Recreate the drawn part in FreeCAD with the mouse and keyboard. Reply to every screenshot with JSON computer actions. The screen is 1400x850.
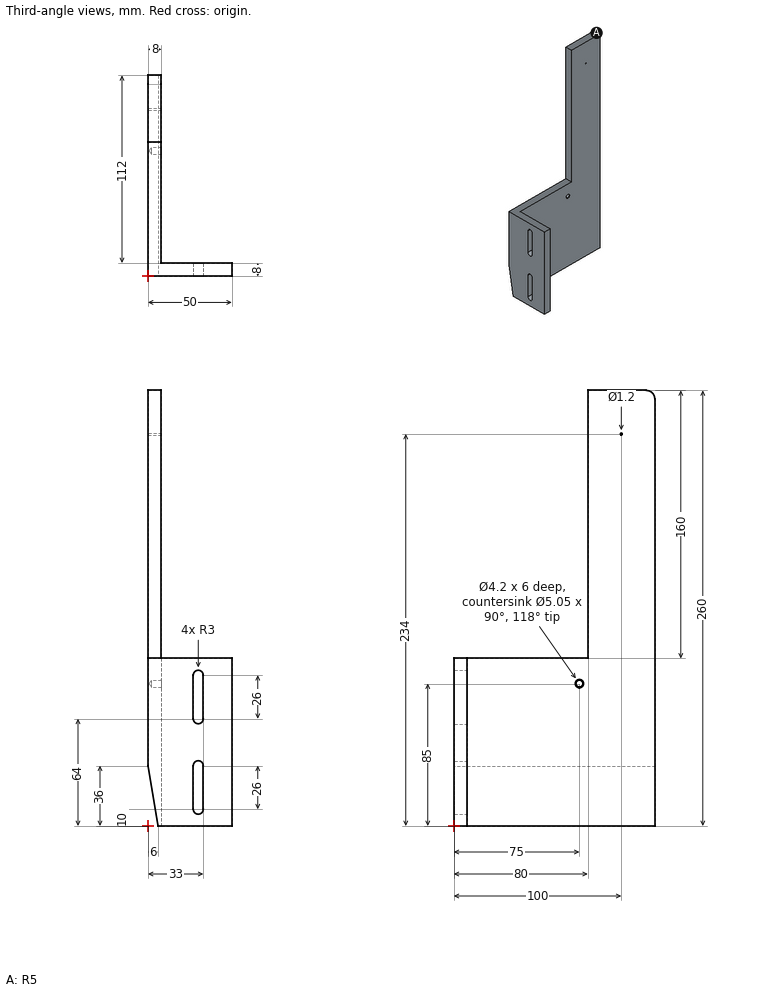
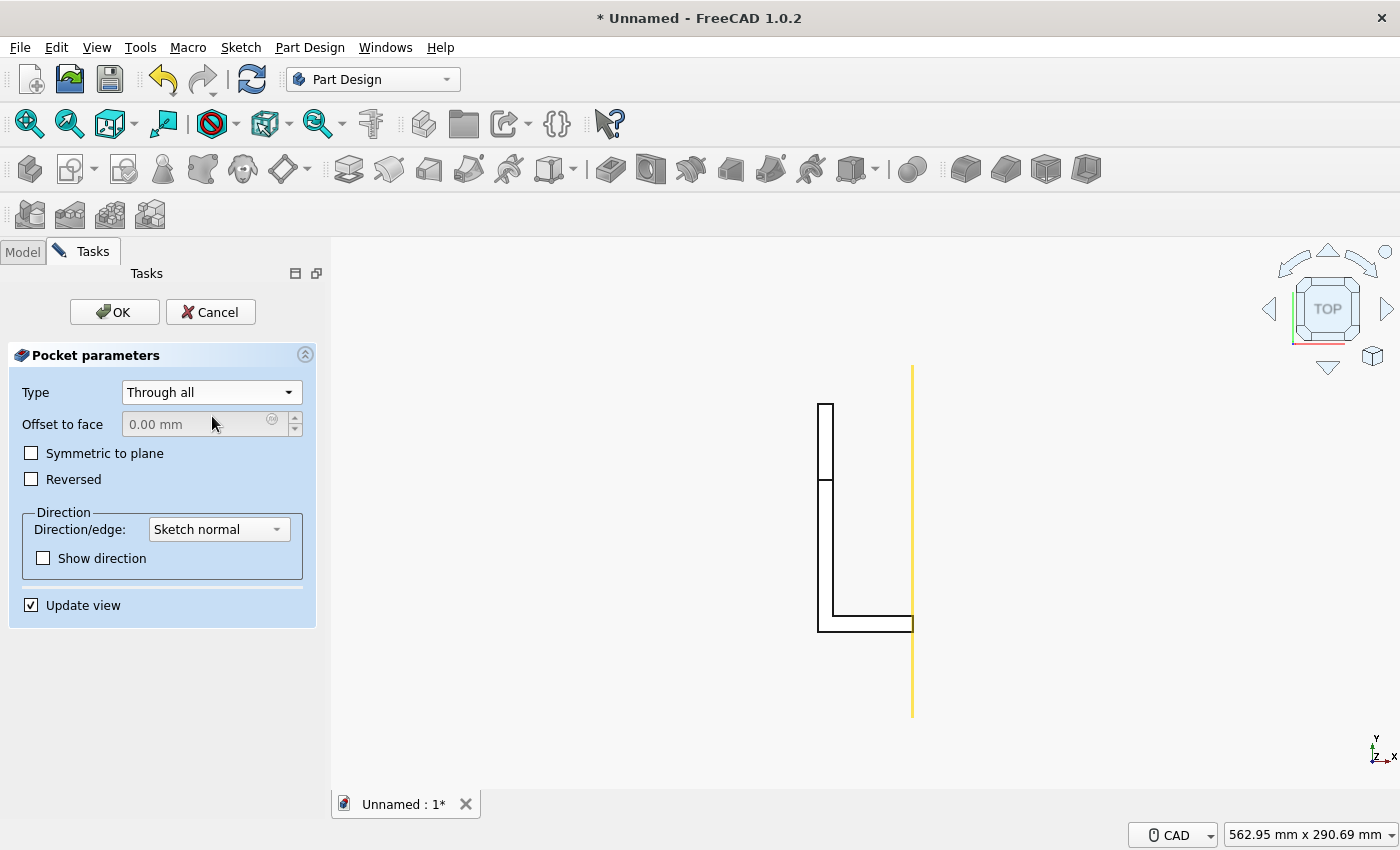
{"action": "left_click", "coordinate": [115, 312]}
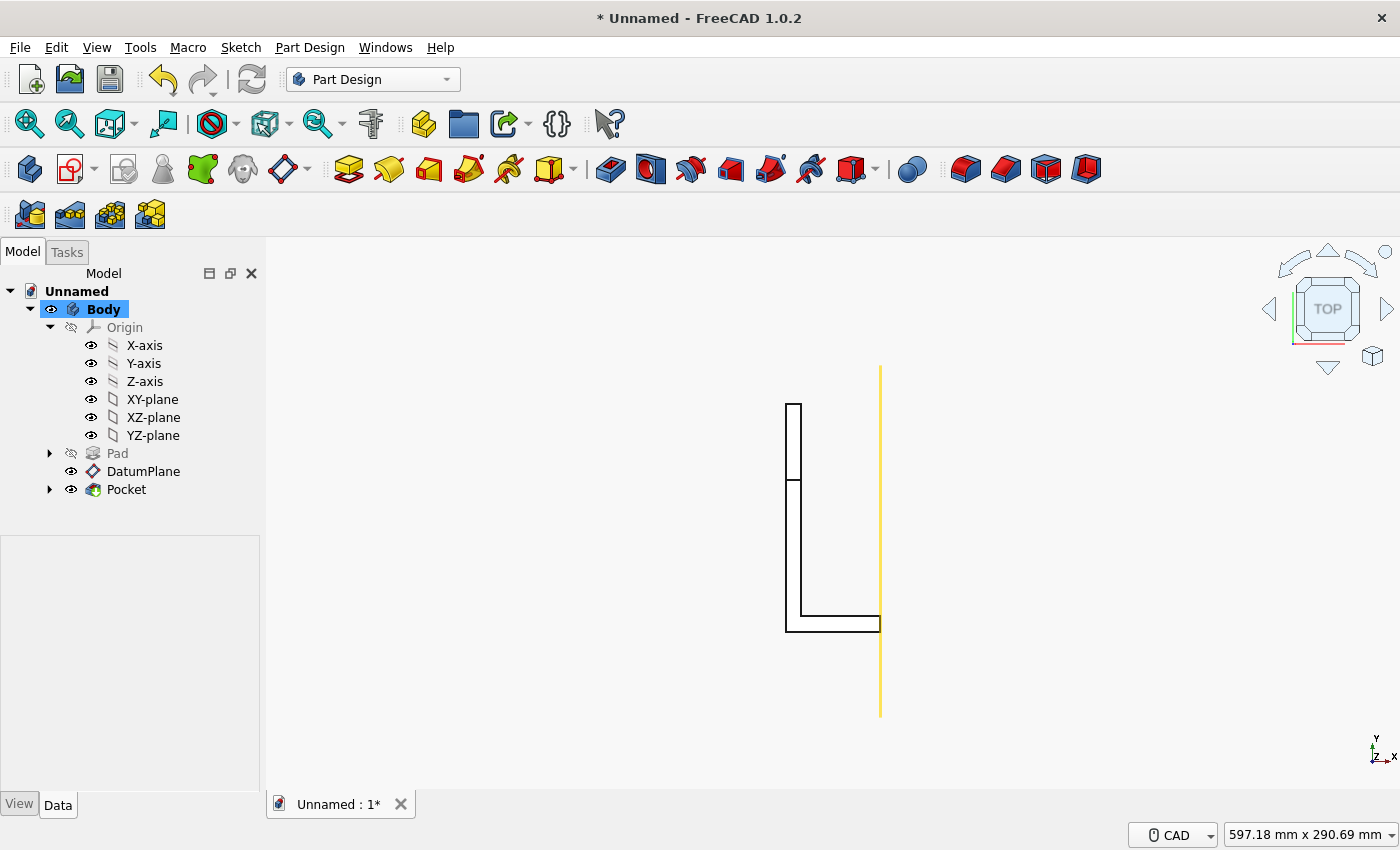
{"action": "left_click", "coordinate": [116, 471]}
{"action": "key", "text": "space"}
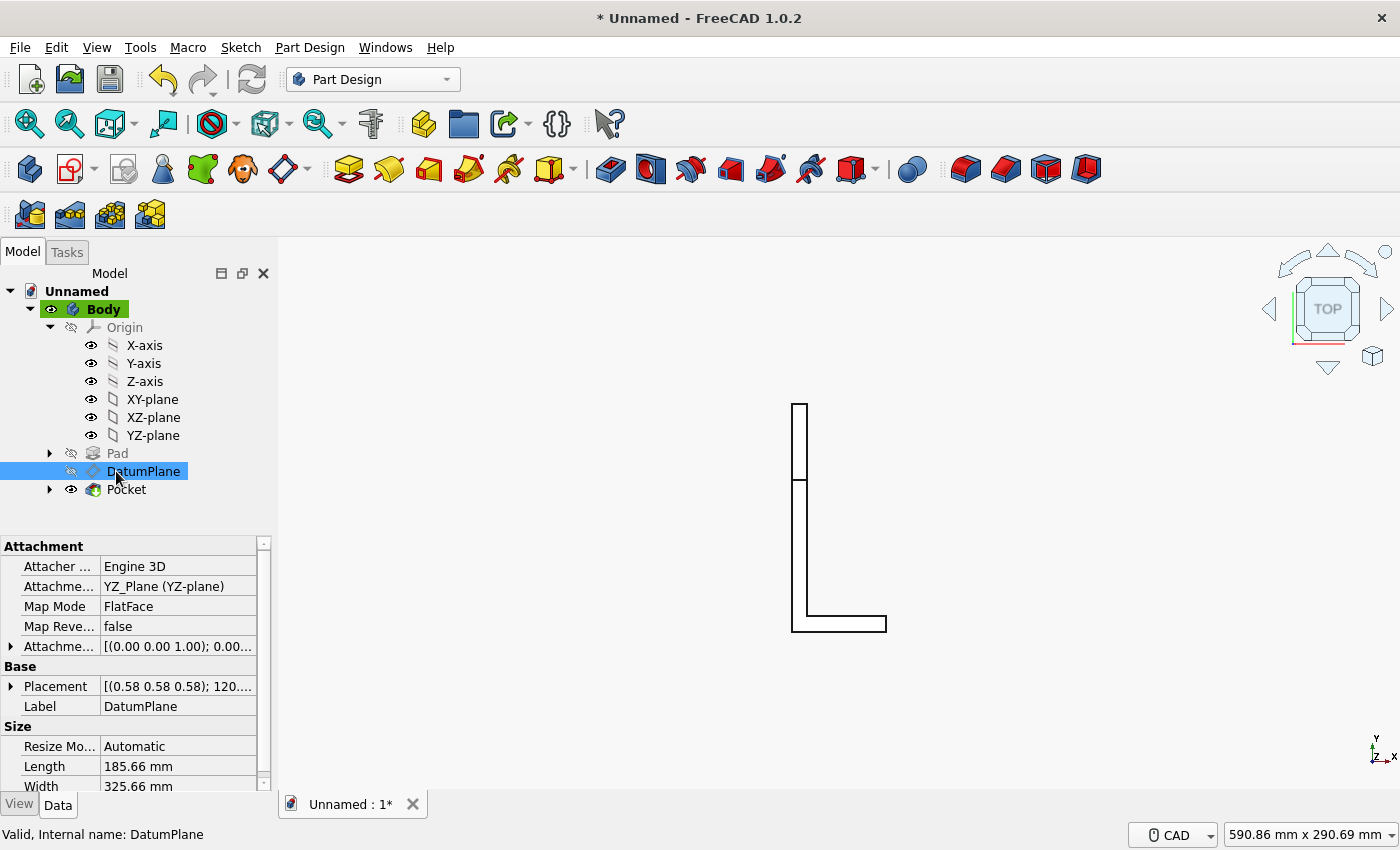
{"action": "left_click", "coordinate": [30, 124]}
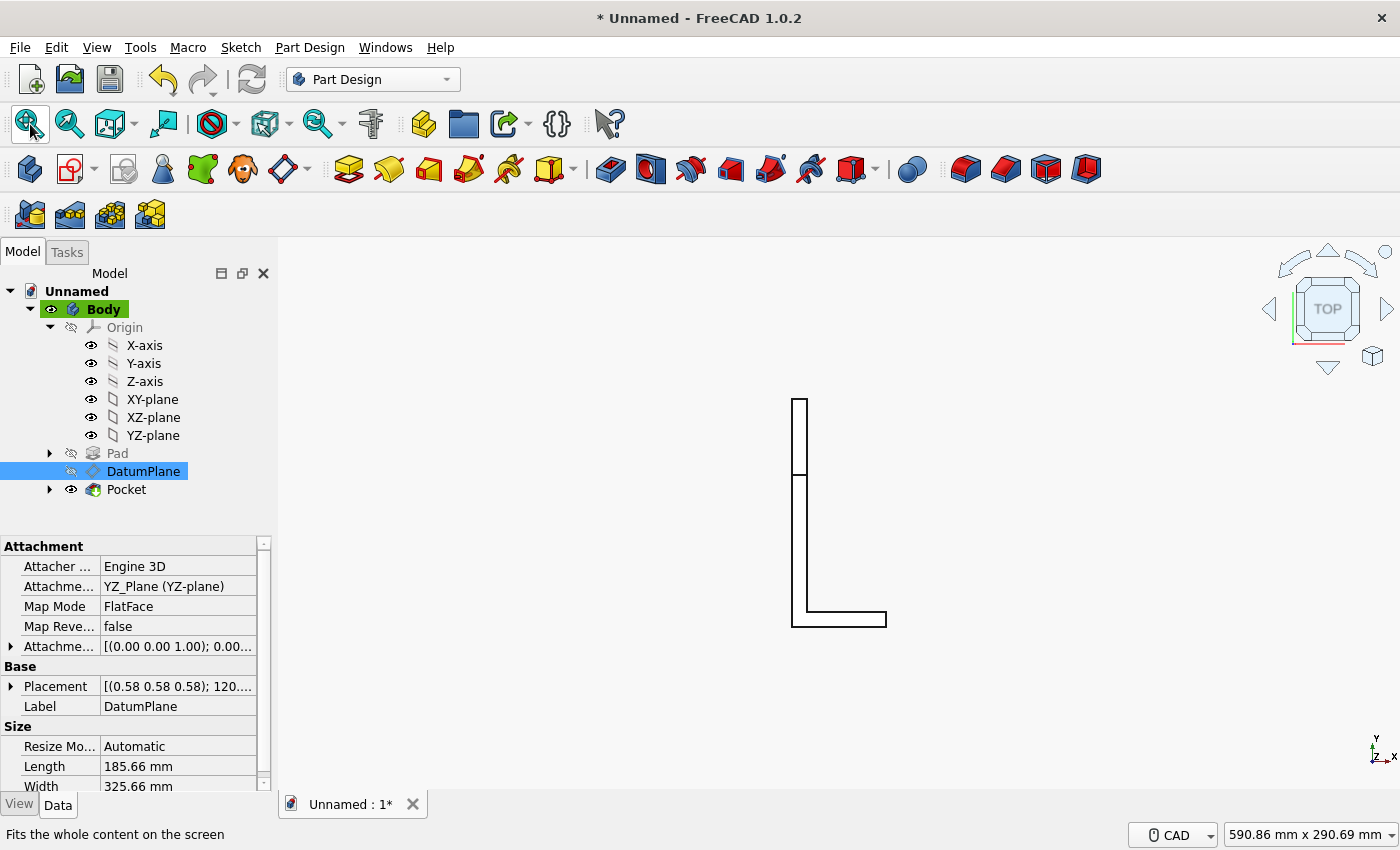
{"action": "key", "text": "4"}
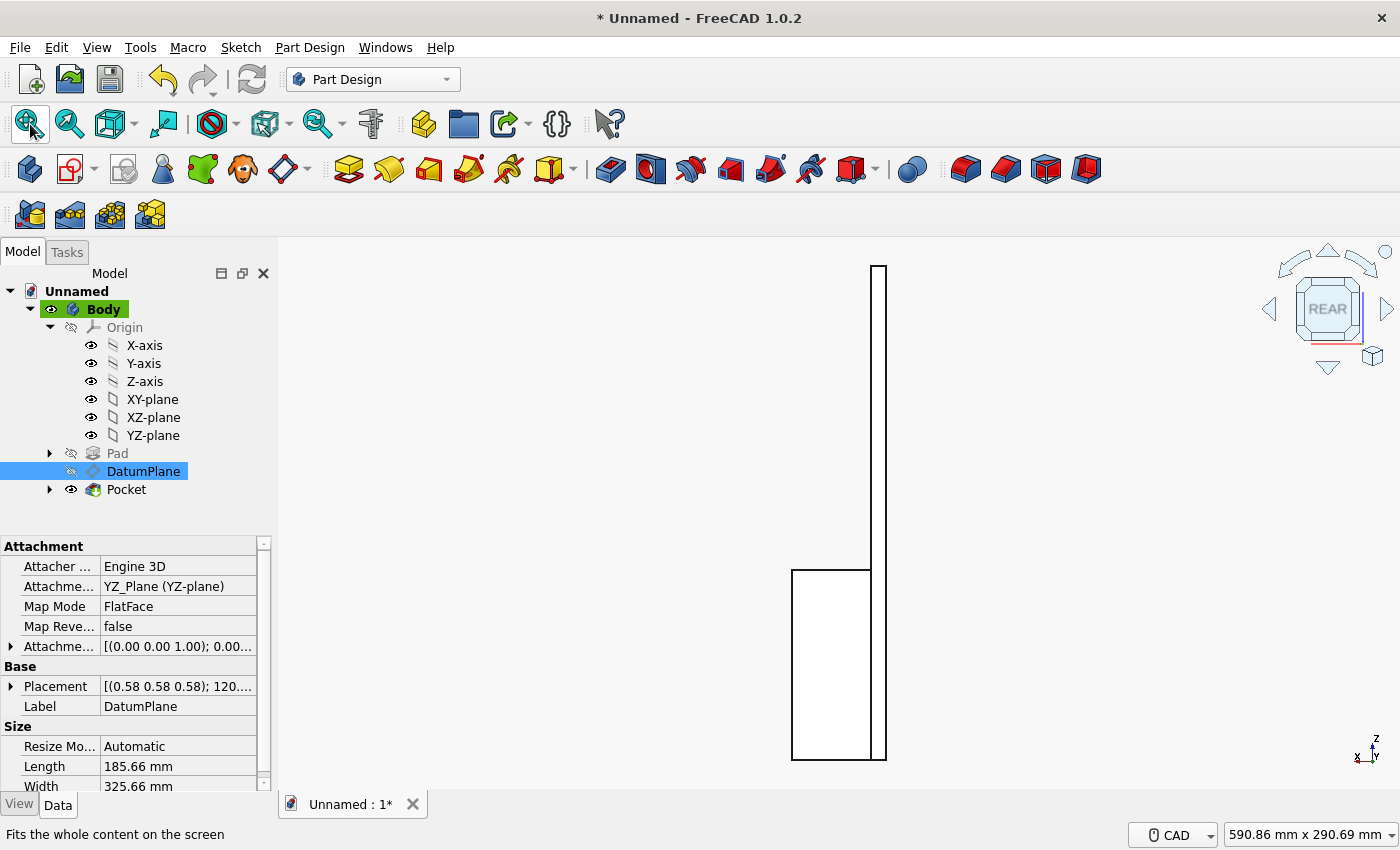
{"action": "left_click", "coordinate": [831, 610]}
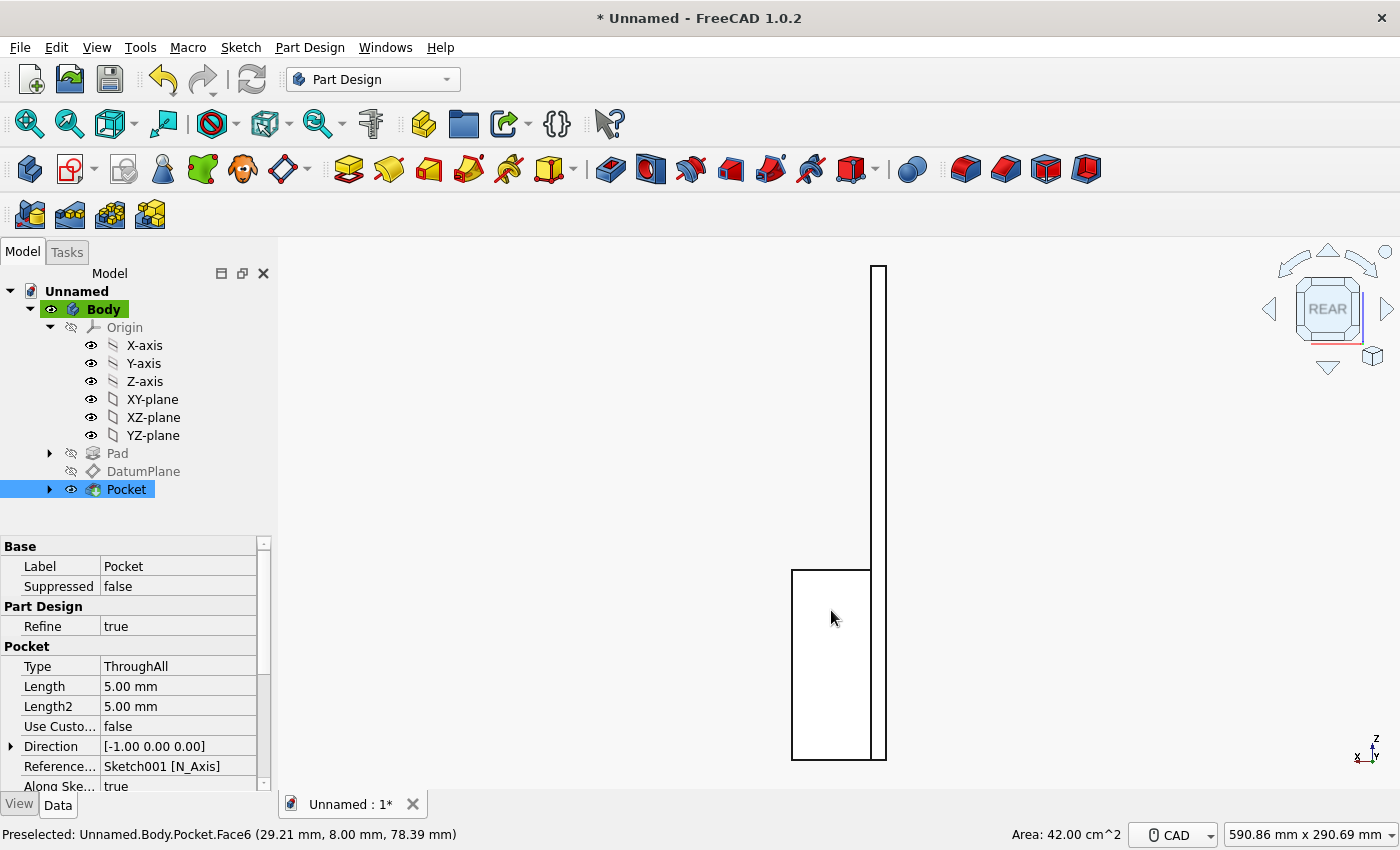
{"action": "left_click", "coordinate": [70, 170]}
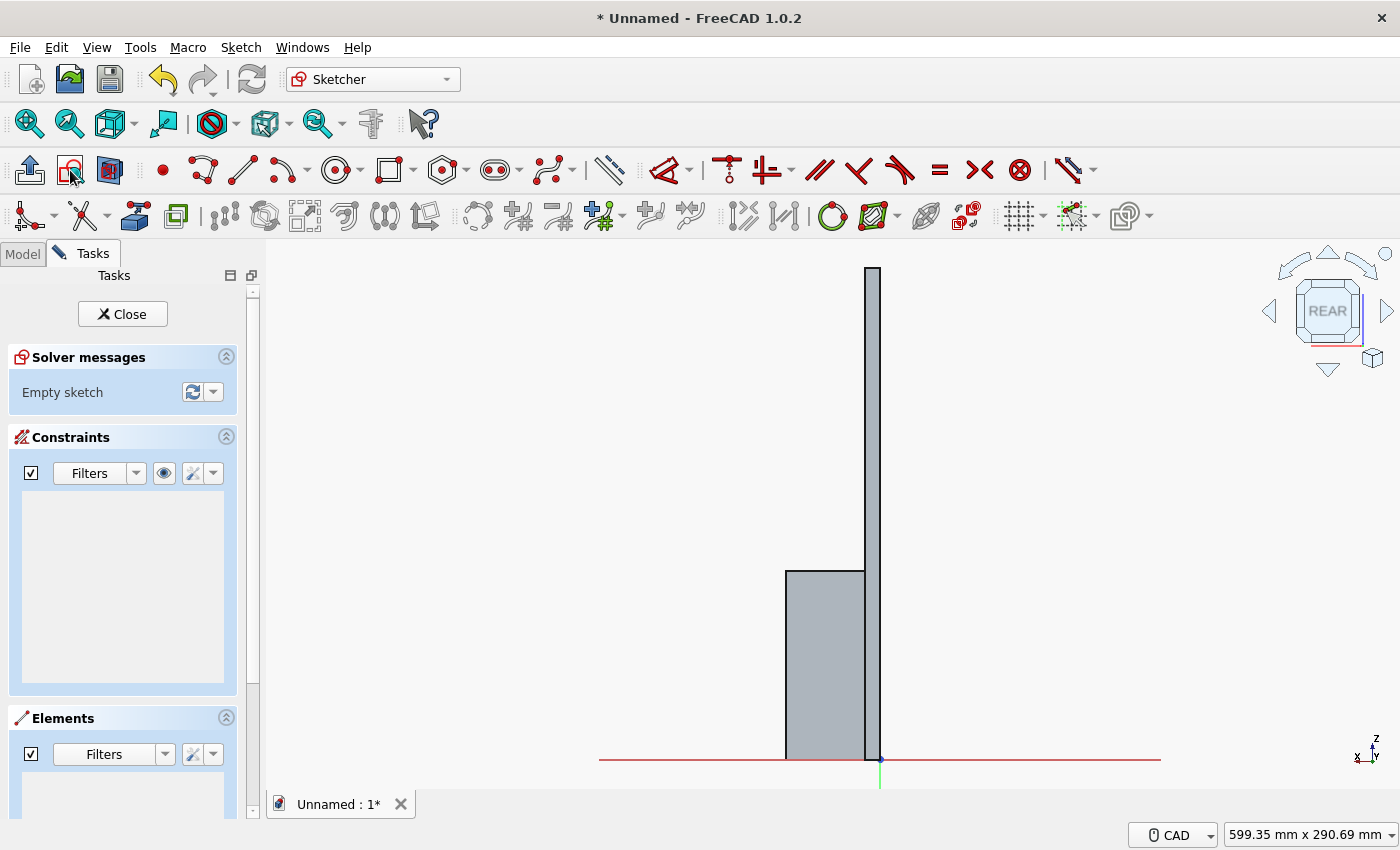
{"action": "left_click", "coordinate": [110, 170]}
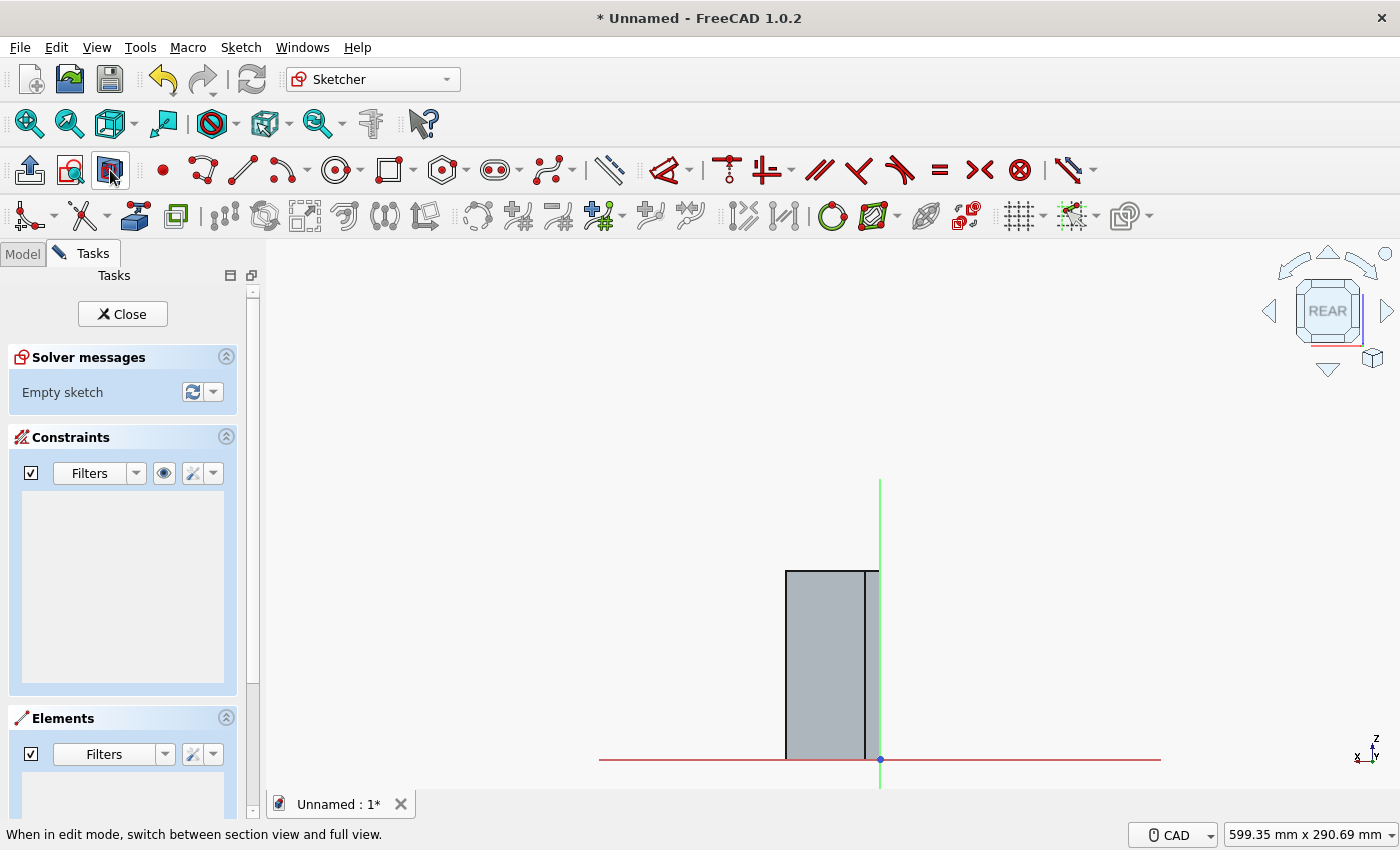
{"action": "scroll", "coordinate": [764, 514], "scroll_direction": "down", "scroll_amount": 5}